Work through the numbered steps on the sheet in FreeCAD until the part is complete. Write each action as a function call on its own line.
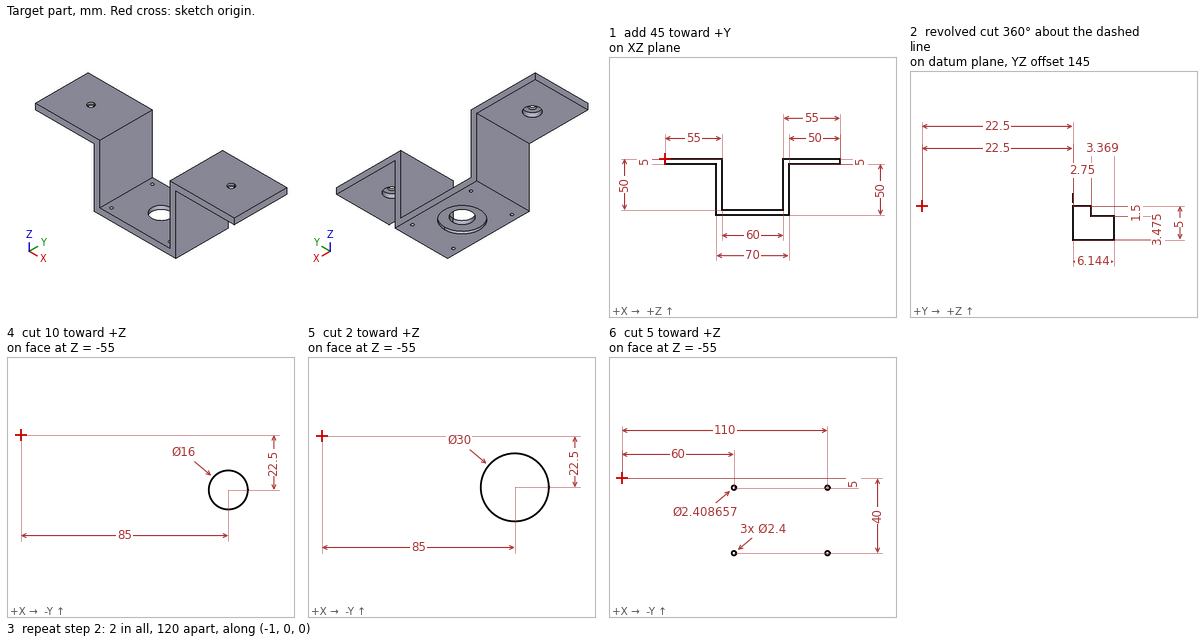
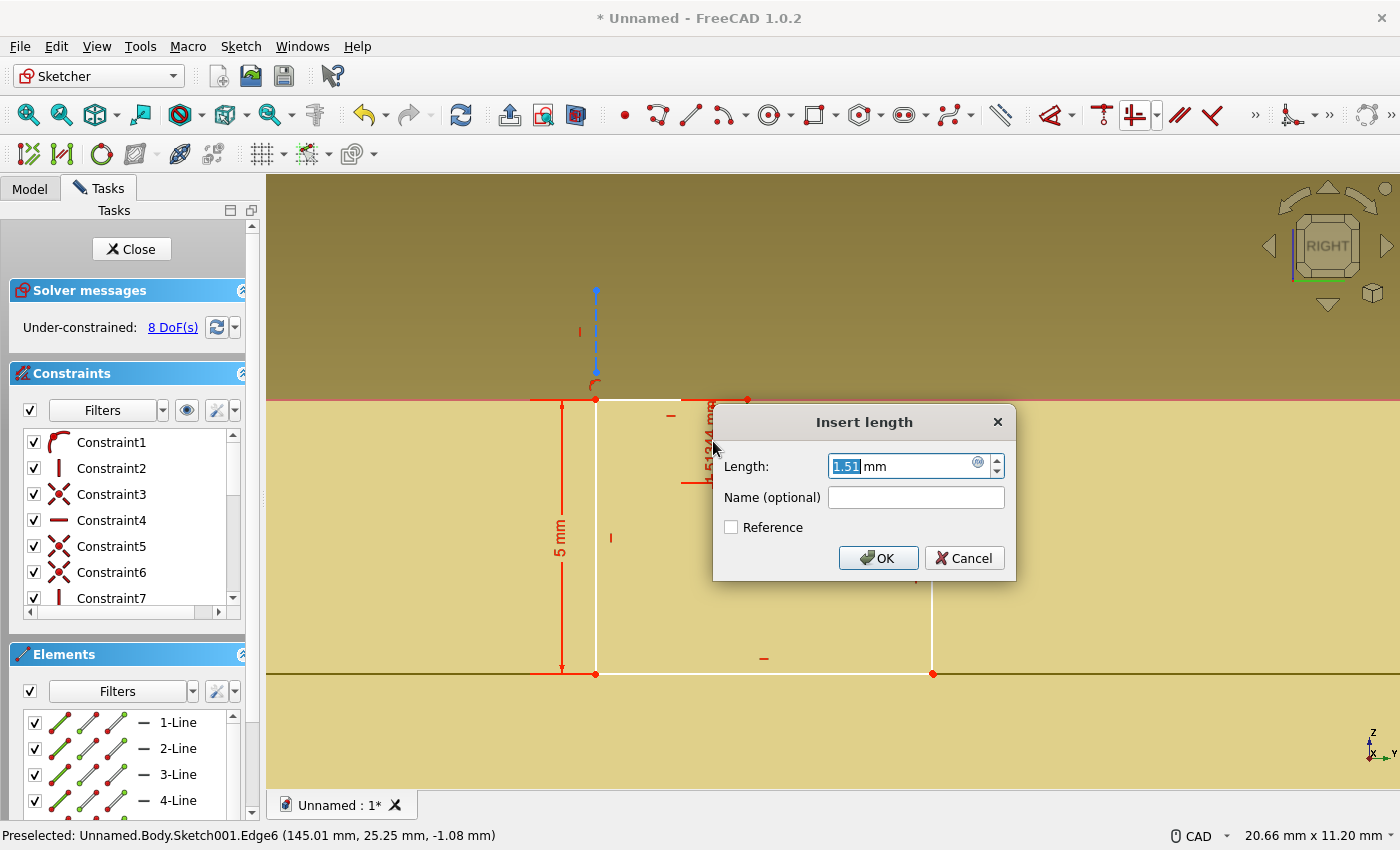
text(1.5)
key(Return)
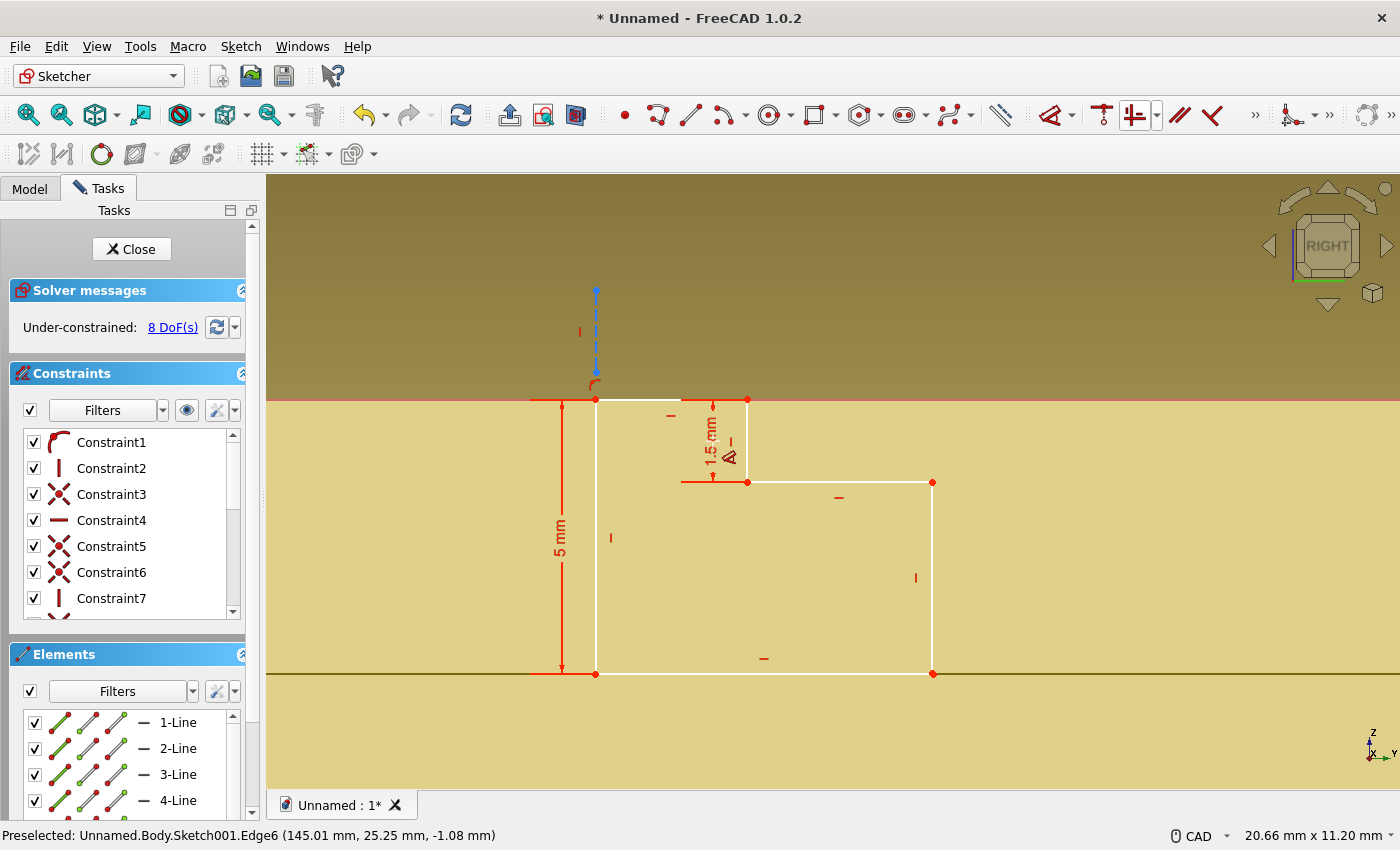
click(702, 400)
click(671, 366)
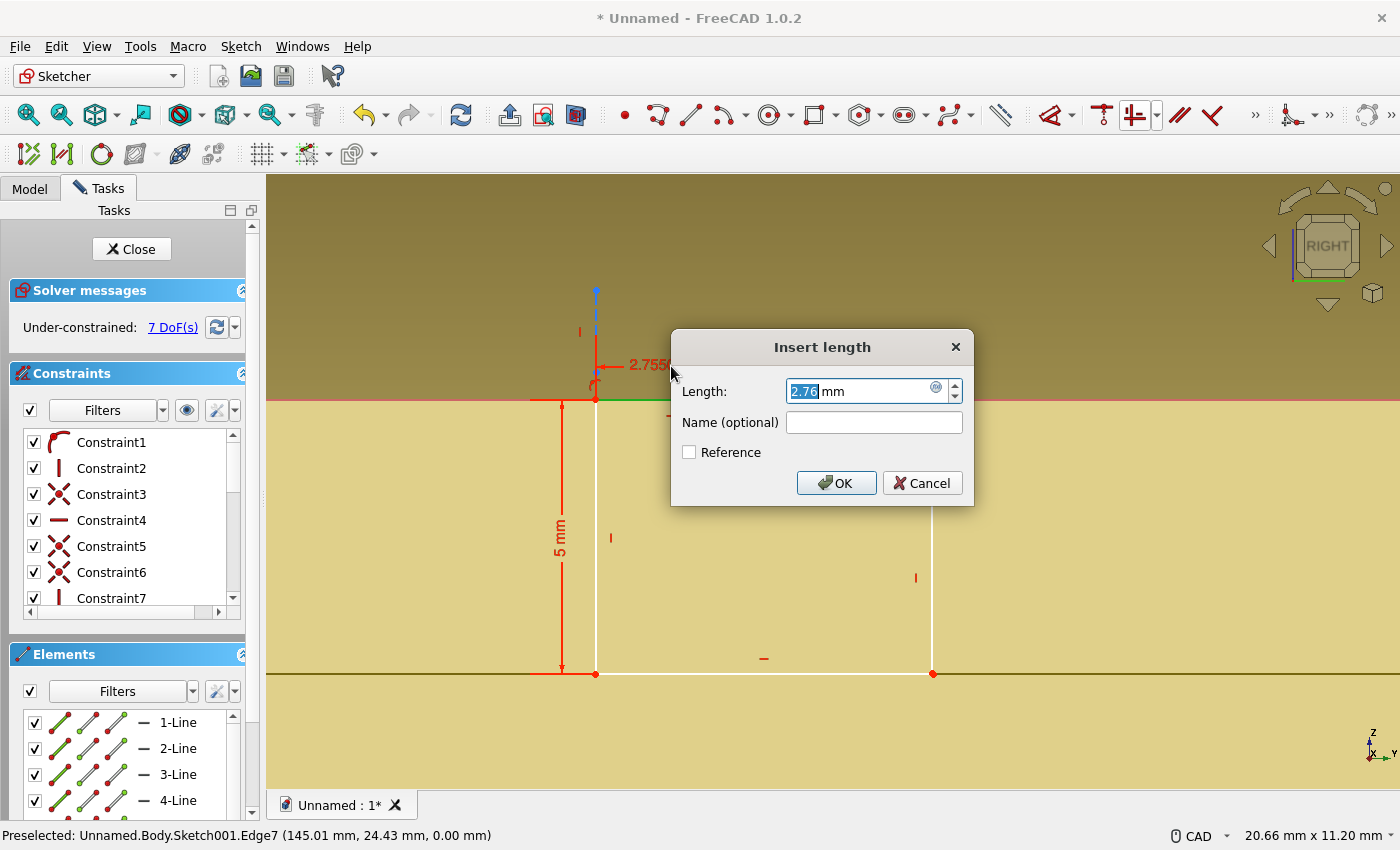
text(2.75)
key(Return)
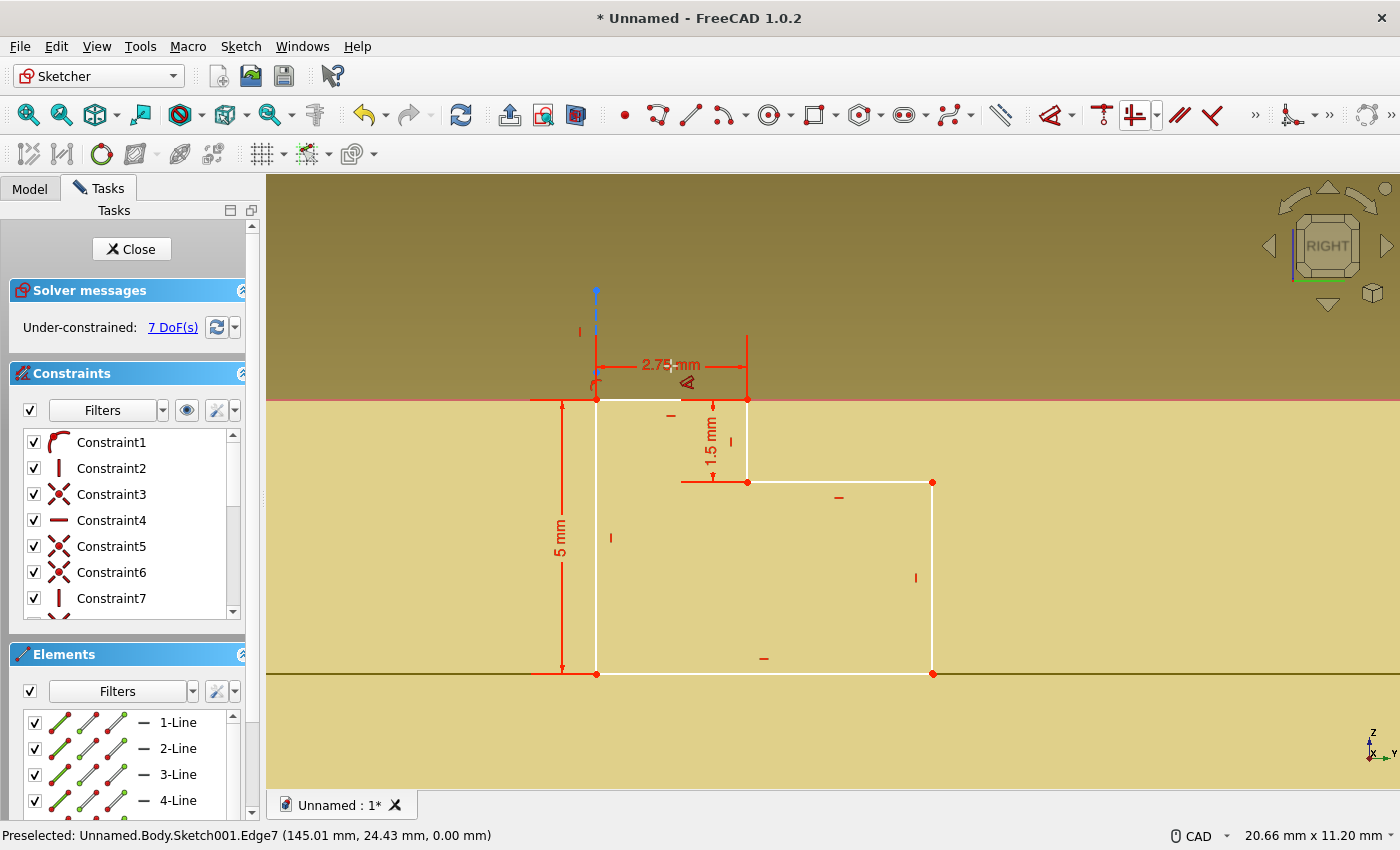
click(697, 674)
click(765, 708)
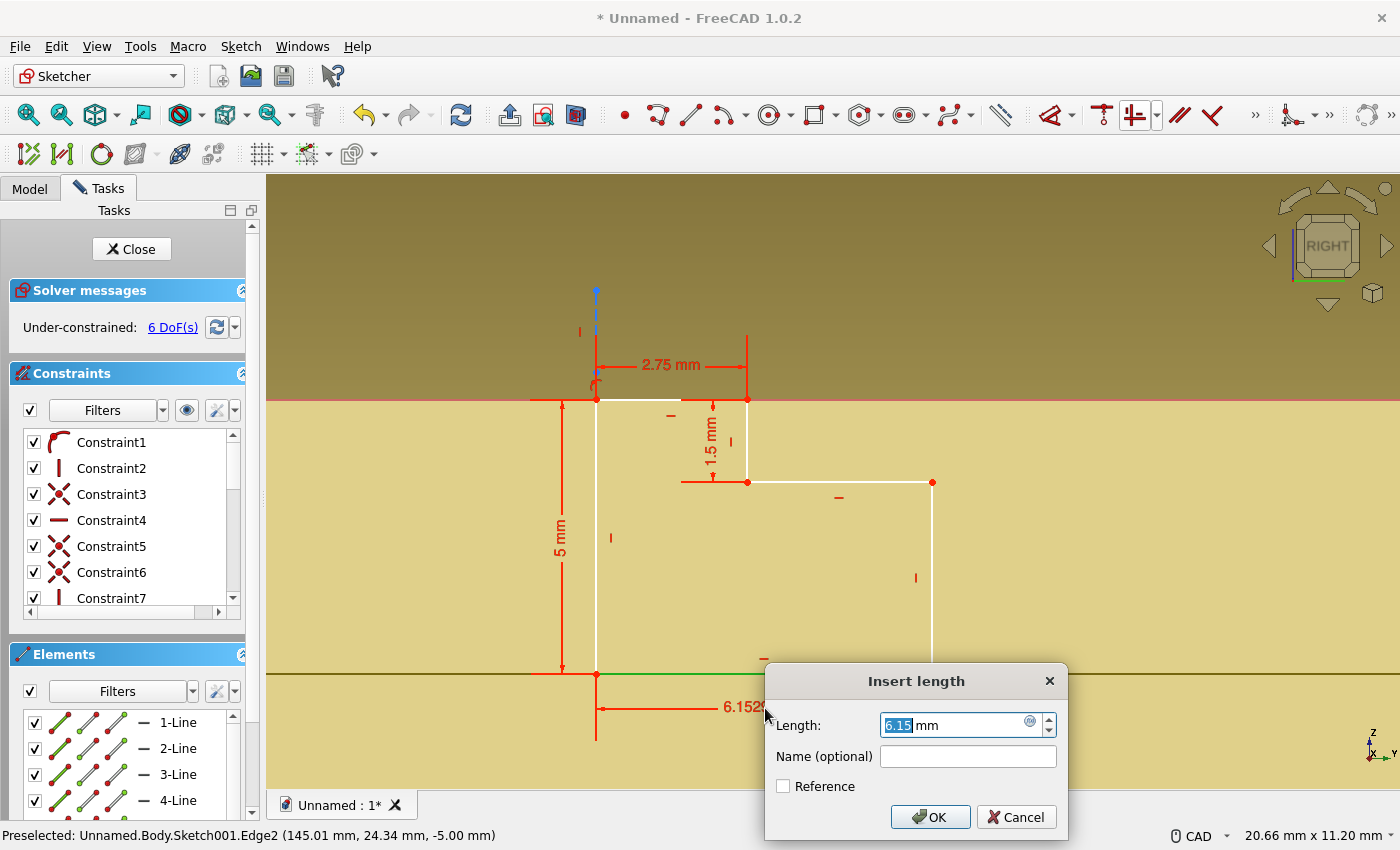
text(6.144)
key(Return)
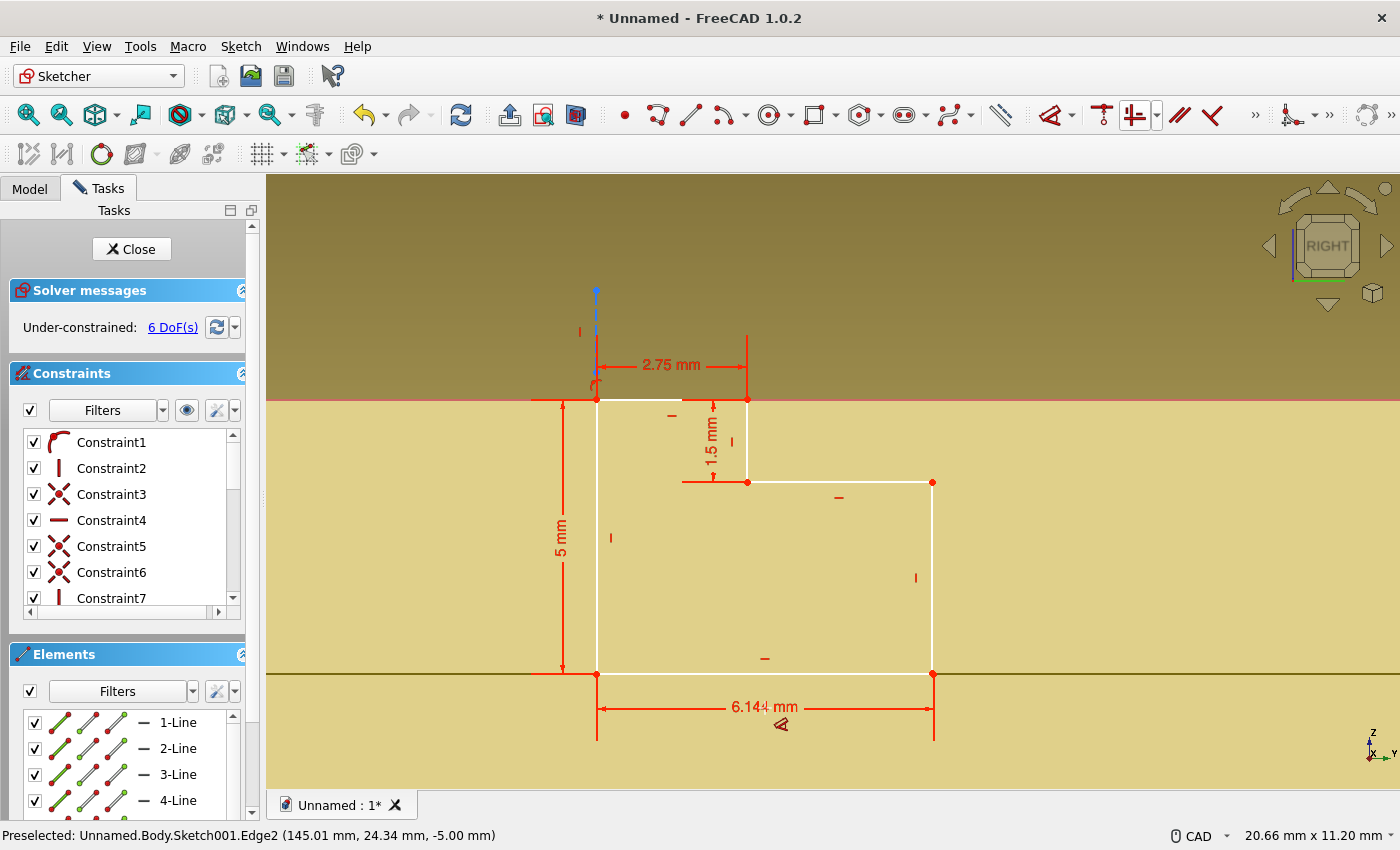
click(932, 616)
click(966, 578)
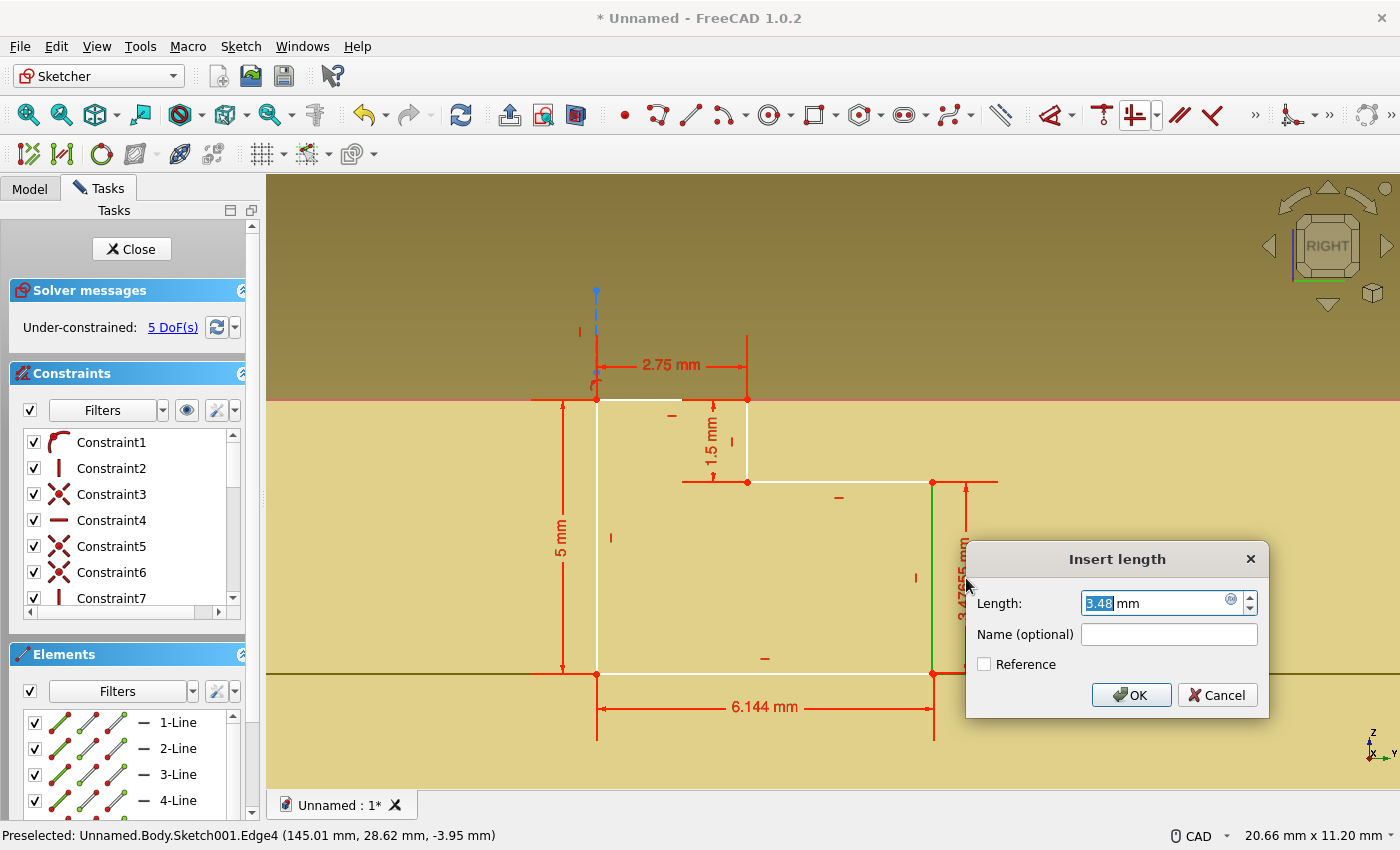
text(3.475)
key(Return)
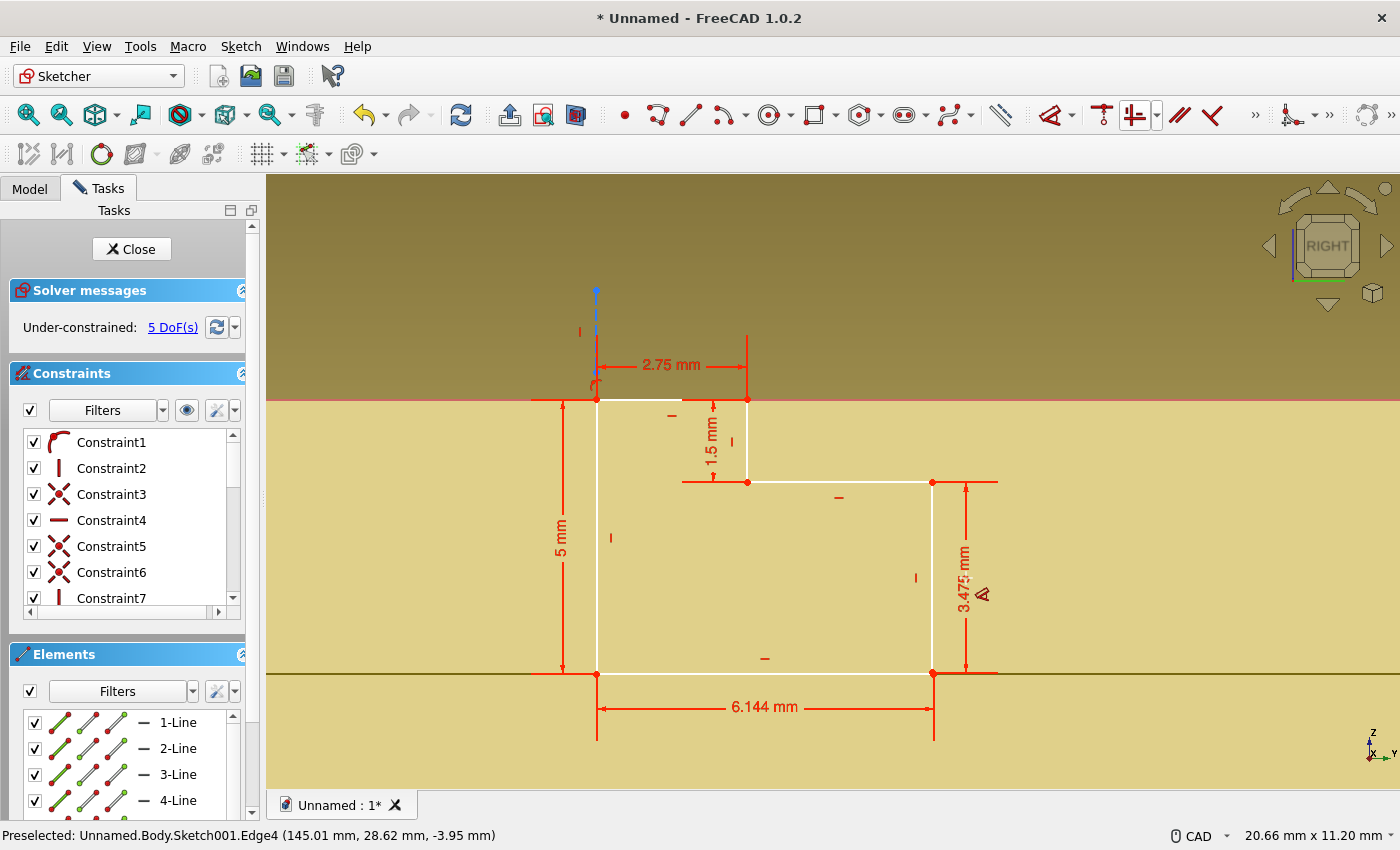
click(877, 482)
click(840, 516)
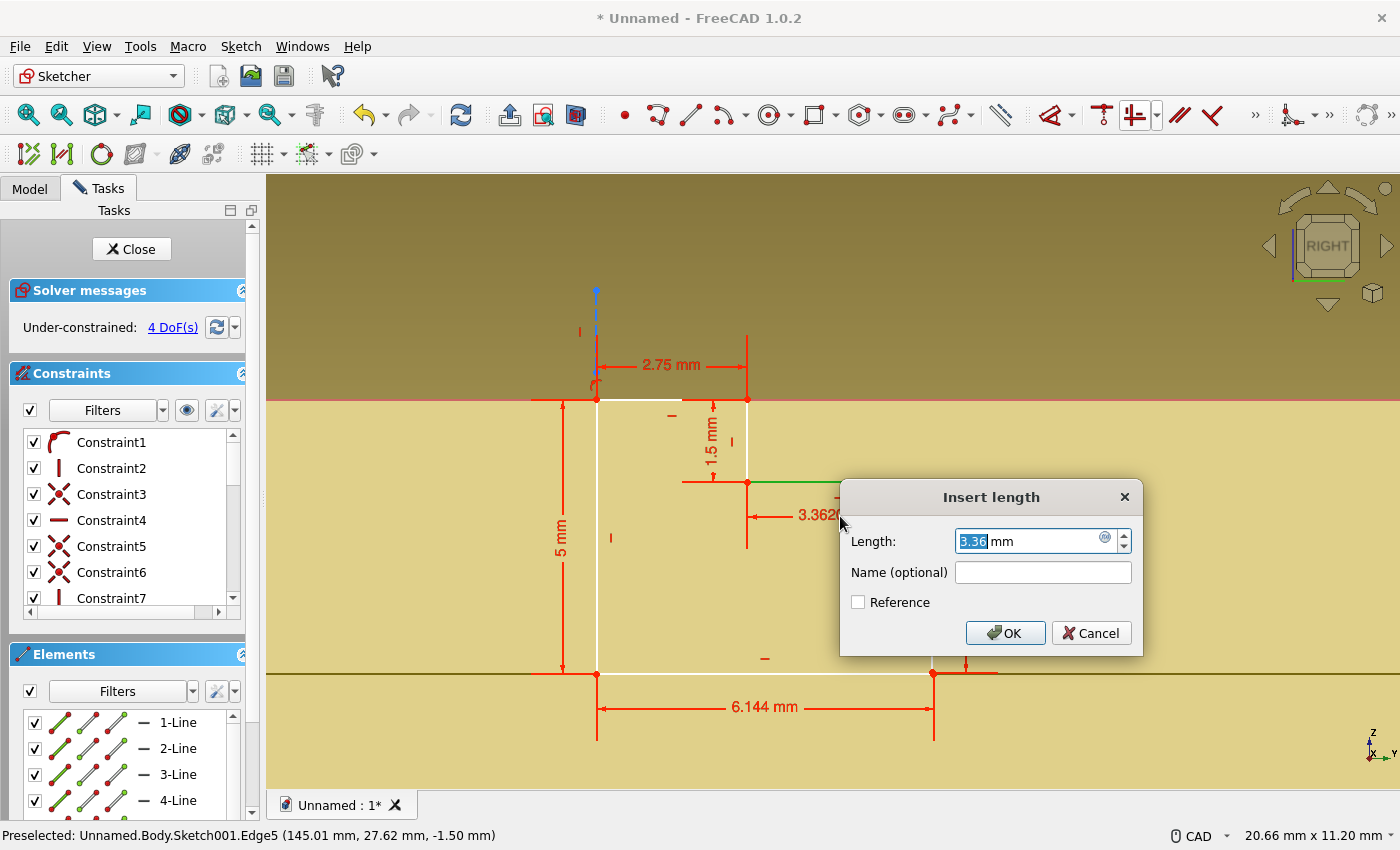
text(3.369)
key(Return)